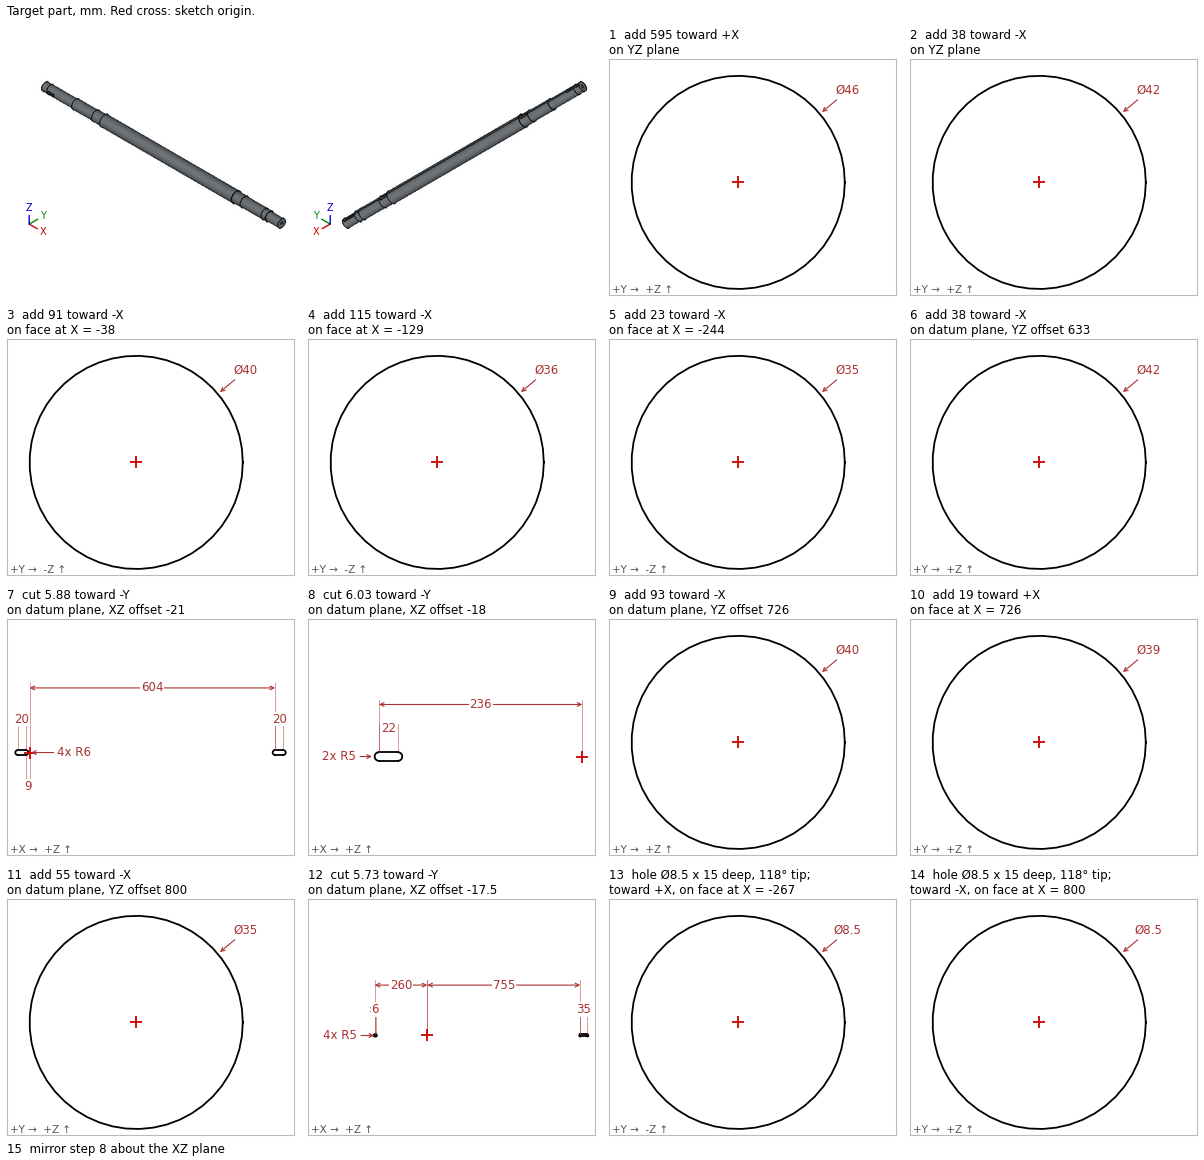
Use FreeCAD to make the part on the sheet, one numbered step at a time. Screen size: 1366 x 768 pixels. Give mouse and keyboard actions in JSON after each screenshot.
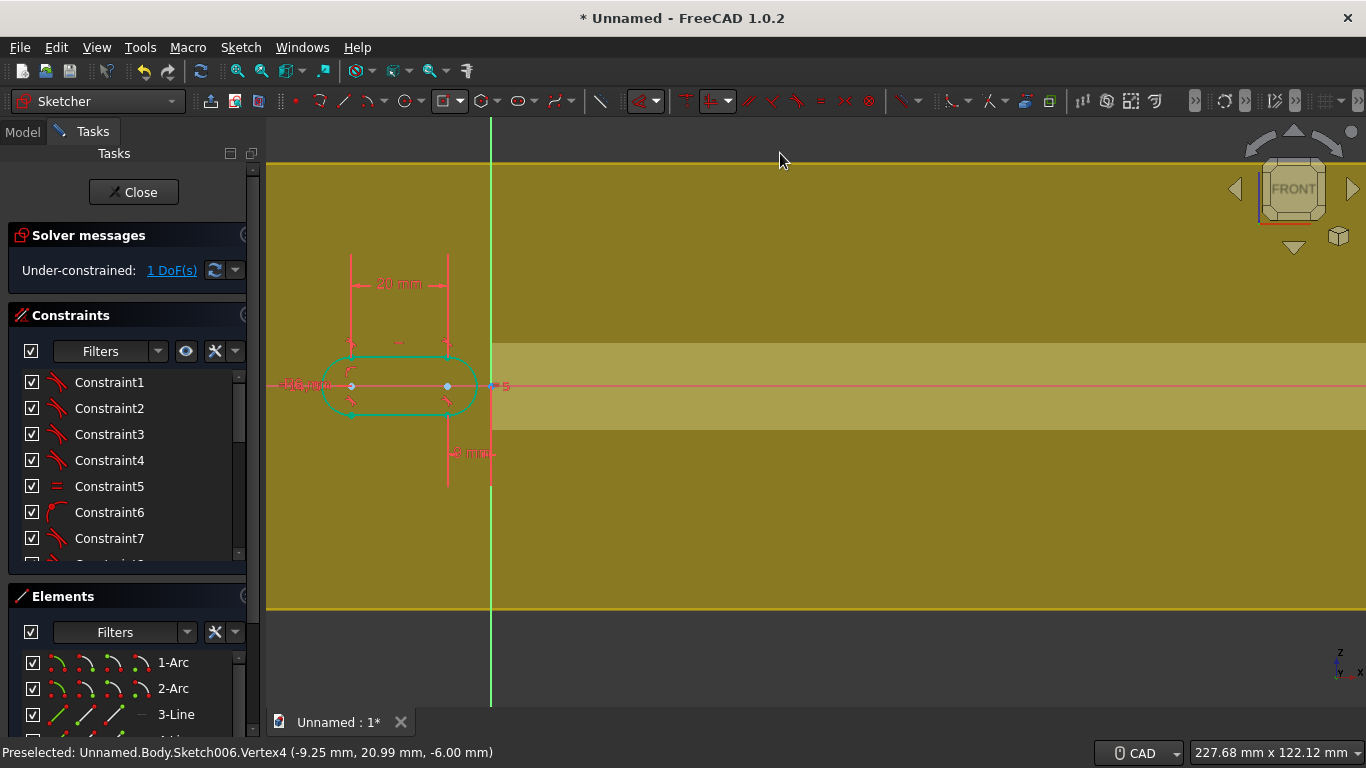
{"action": "scroll", "coordinate": [449, 418], "scroll_direction": "down", "scroll_amount": 8}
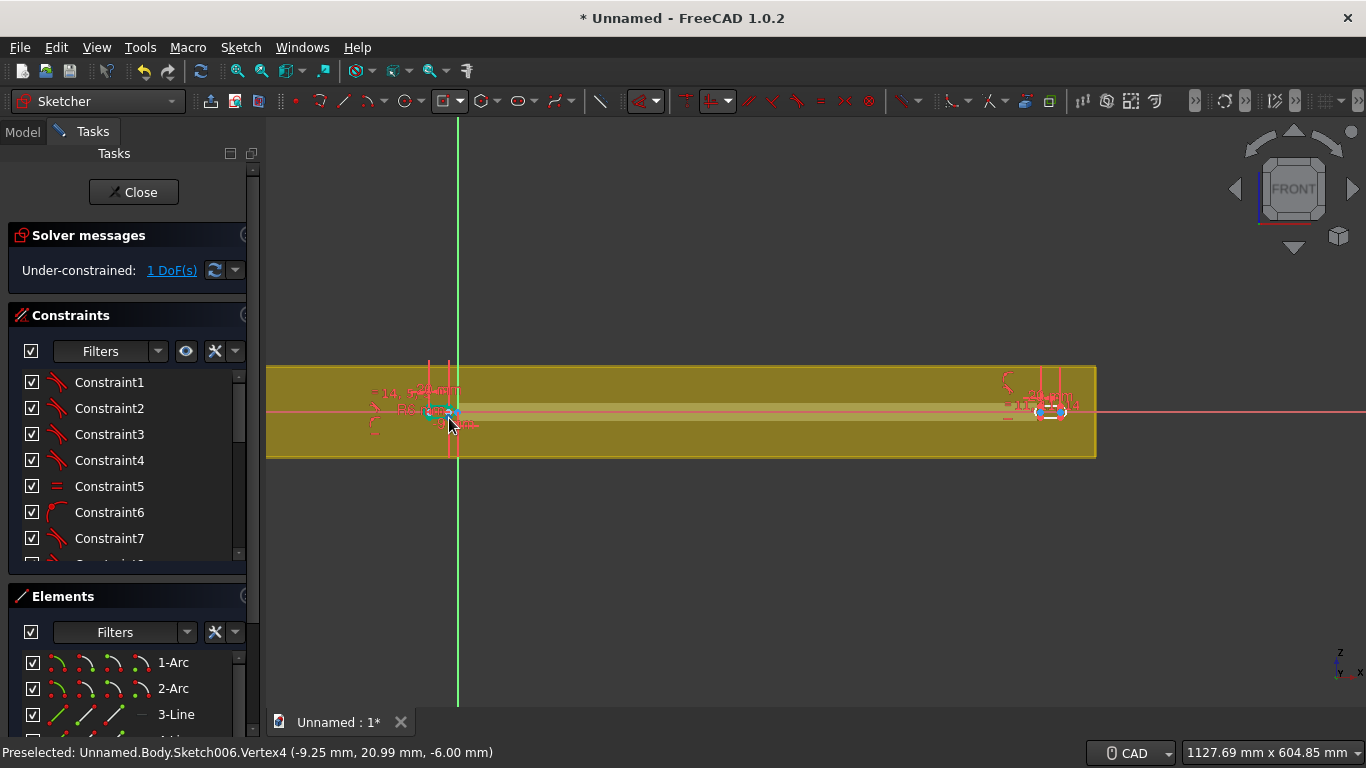
{"action": "scroll", "coordinate": [1041, 406], "scroll_direction": "up", "scroll_amount": 4}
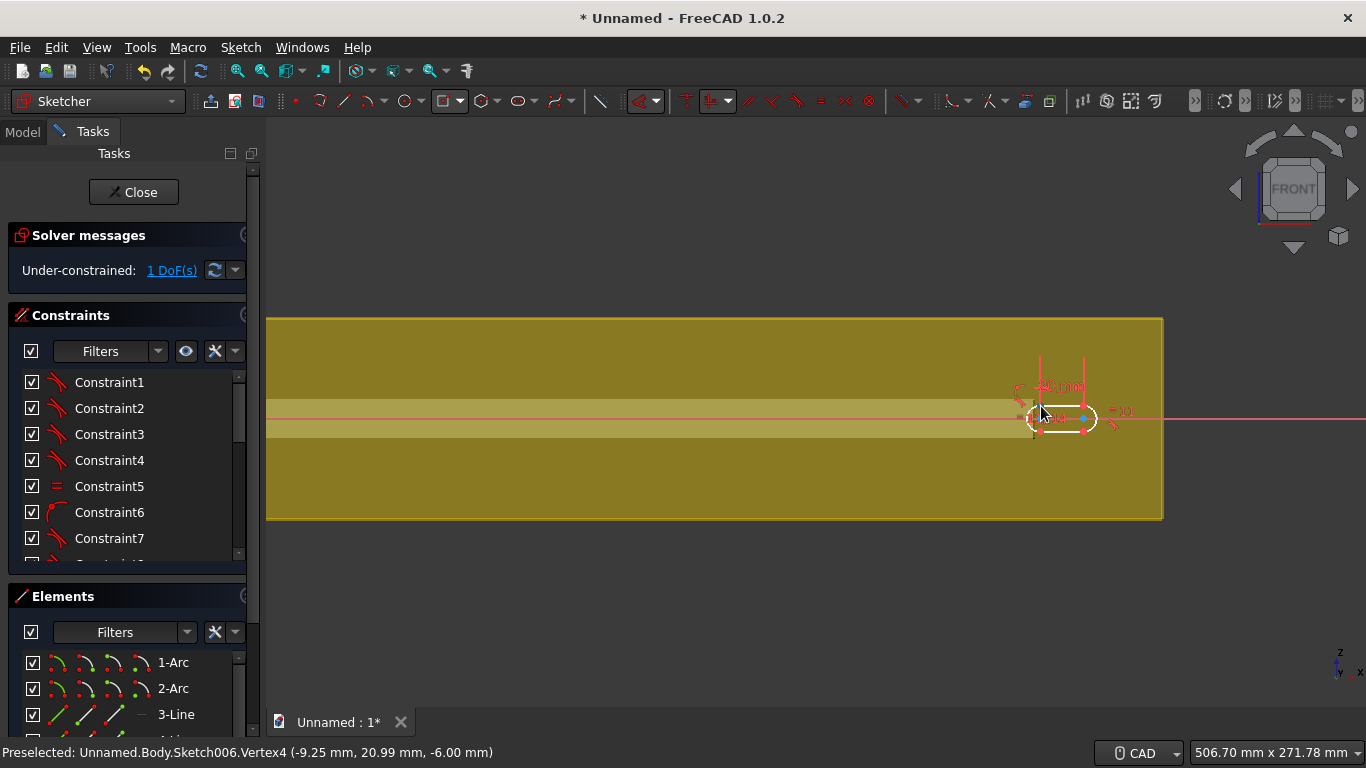
{"action": "left_click", "coordinate": [1040, 406]}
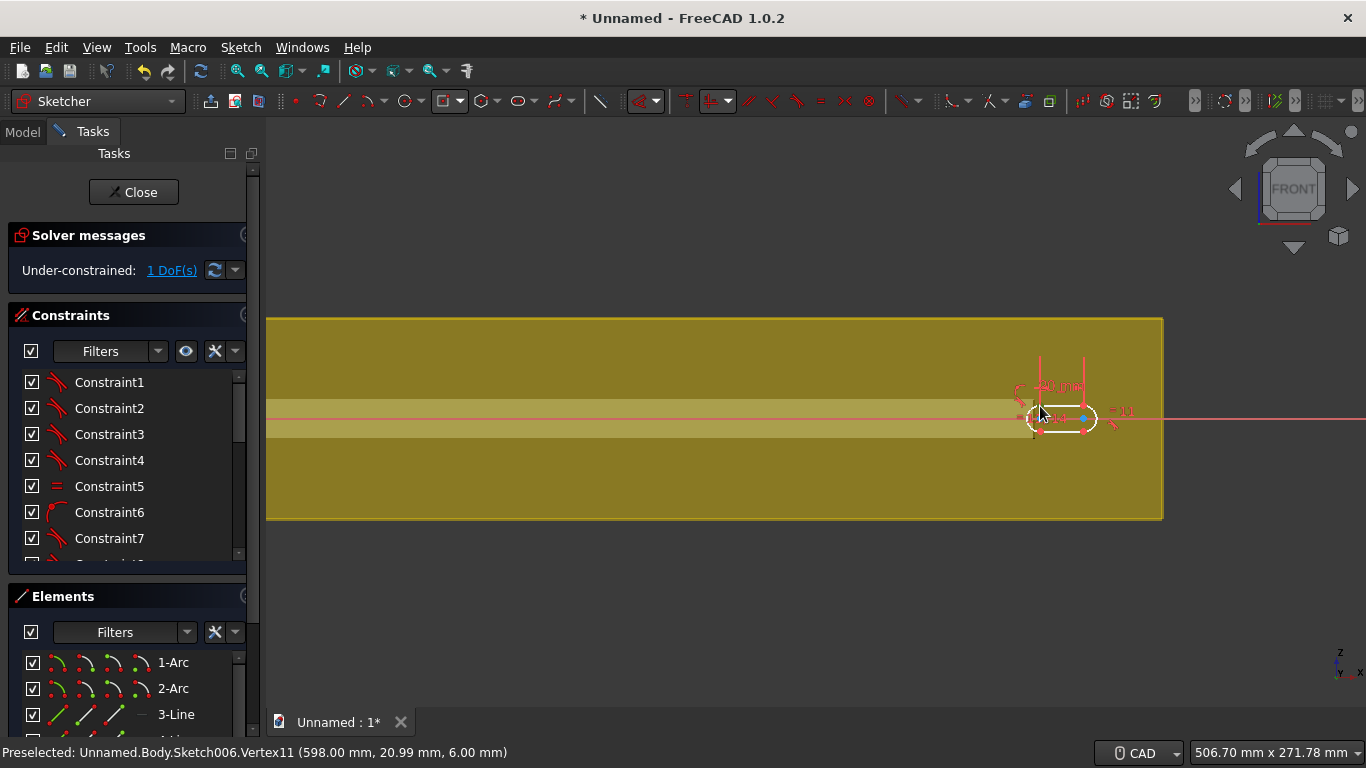
{"action": "left_click", "coordinate": [658, 102]}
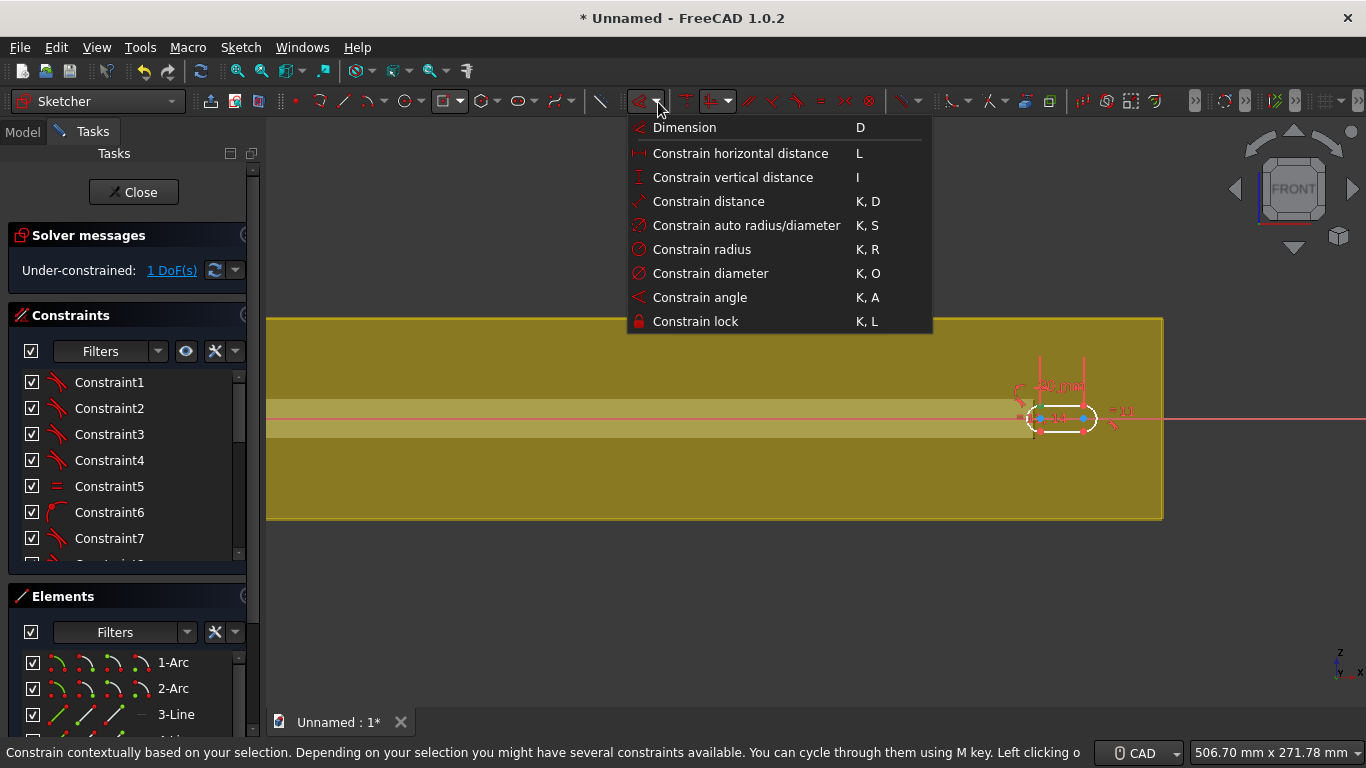
{"action": "left_click", "coordinate": [780, 153]}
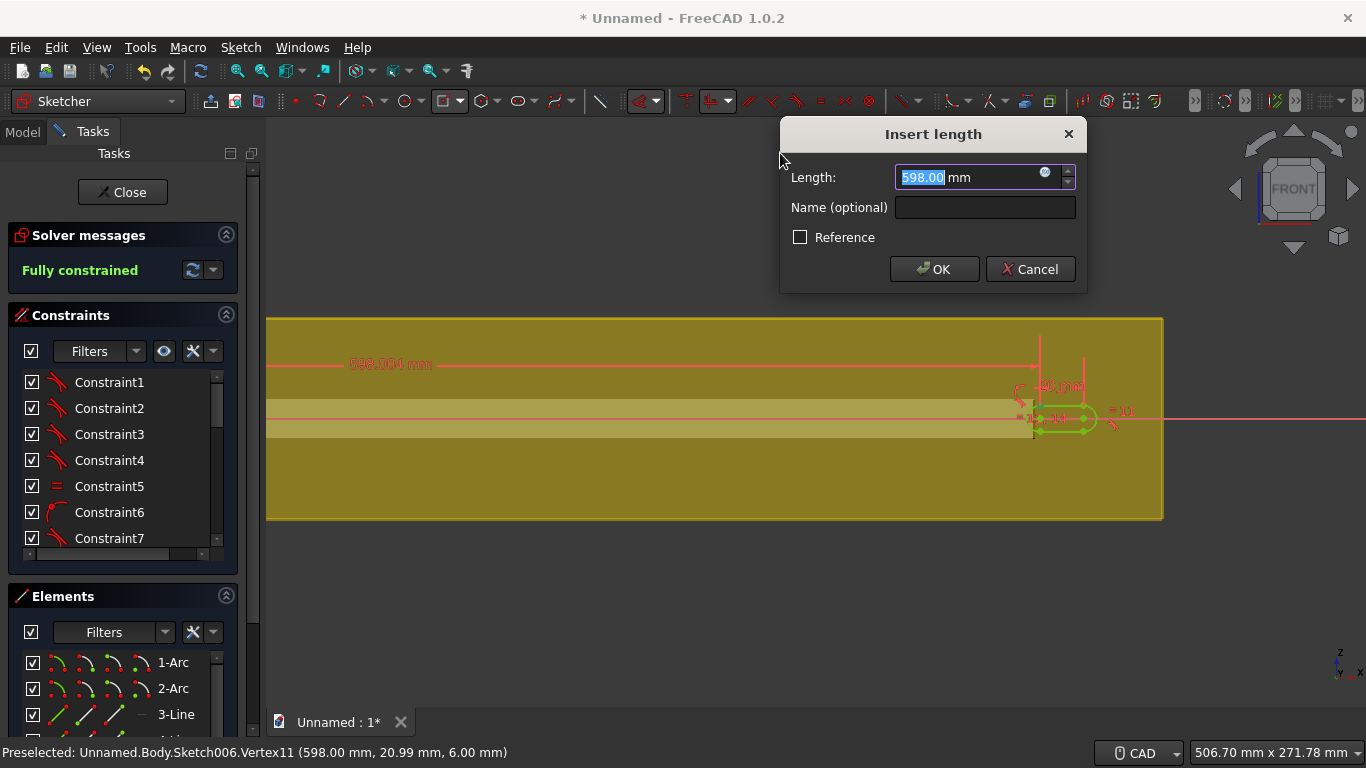
{"action": "type", "text": "604"}
{"action": "key", "text": "Return"}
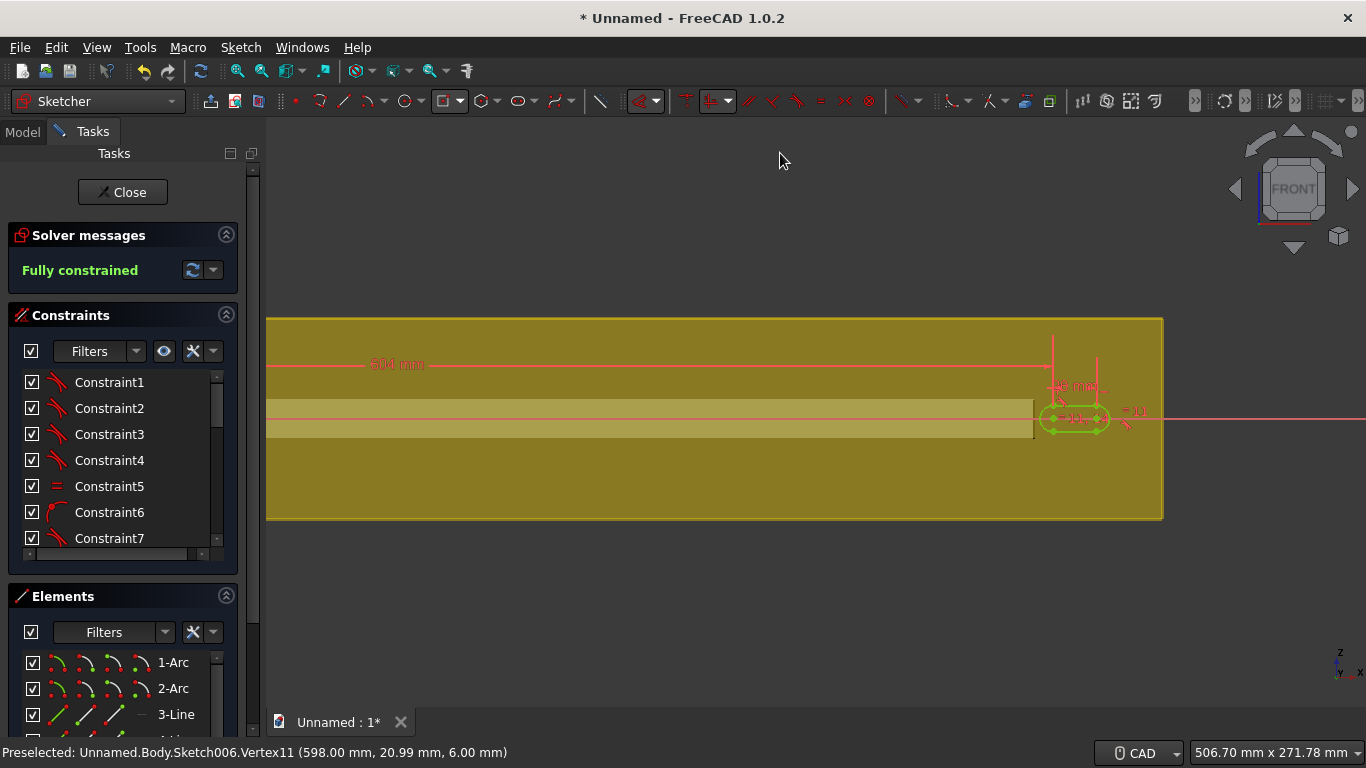
{"action": "left_click", "coordinate": [123, 192]}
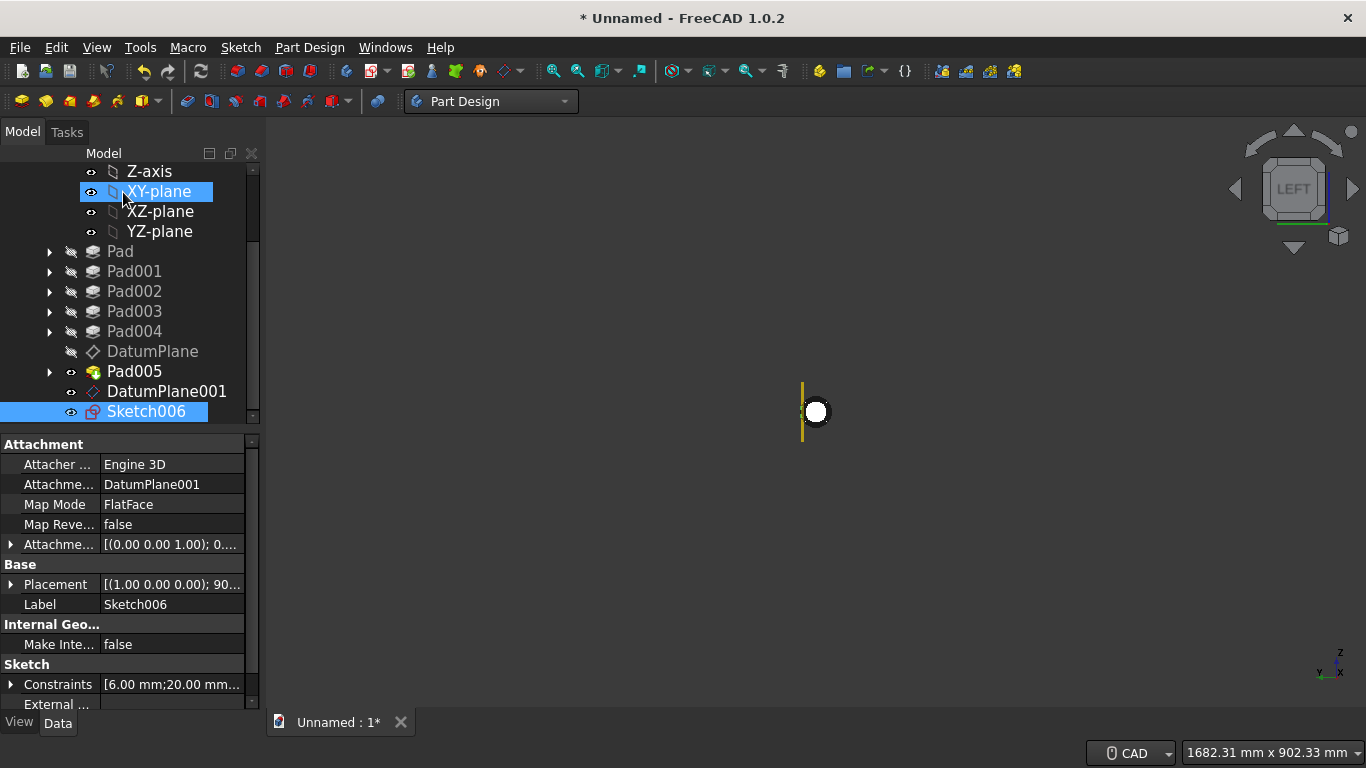
{"action": "left_click", "coordinate": [188, 102]}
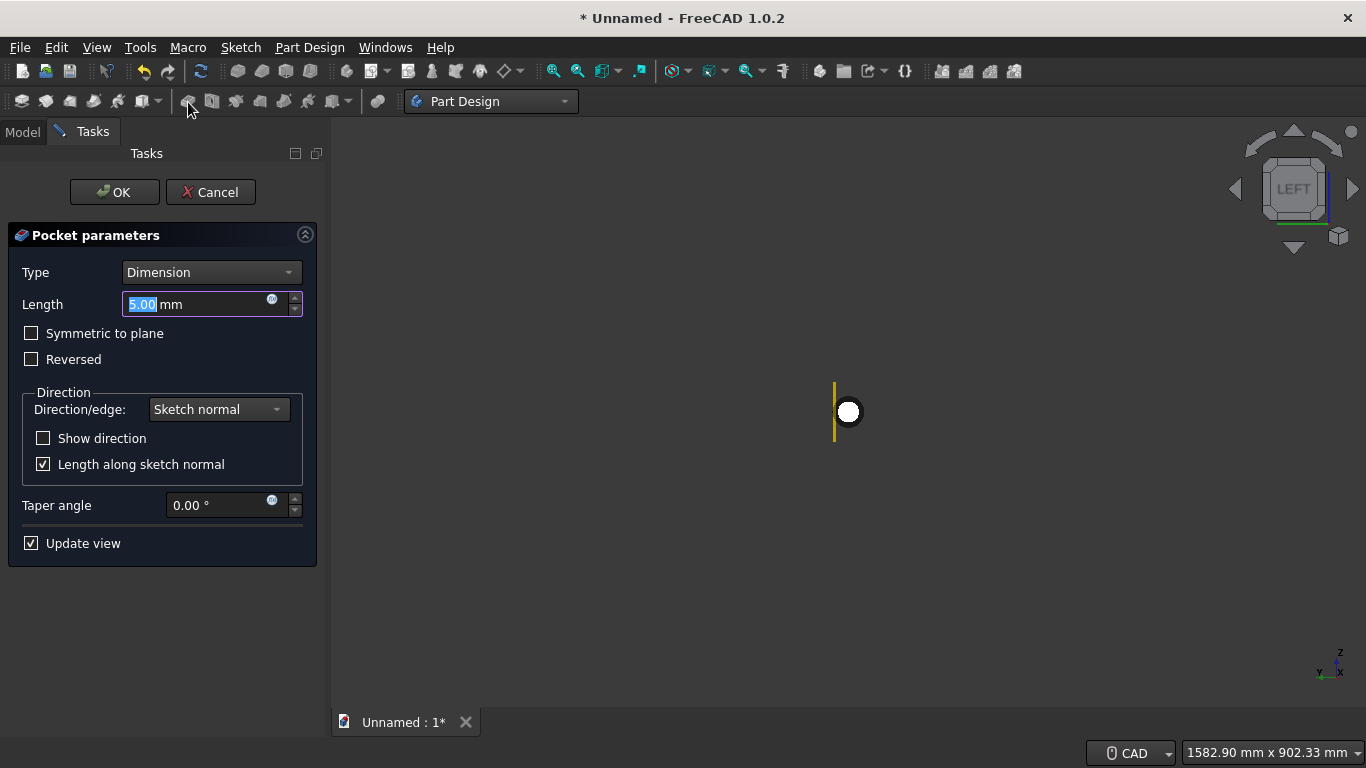
{"action": "type", "text": "5.88"}
{"action": "key", "text": "Tab"}